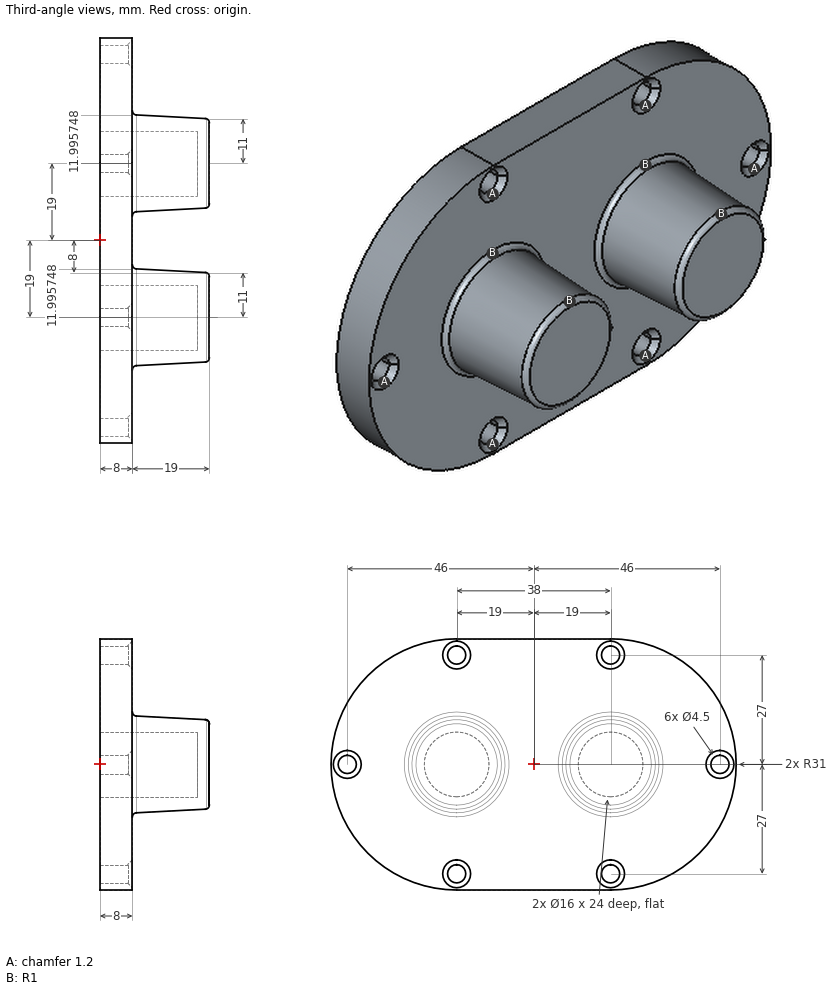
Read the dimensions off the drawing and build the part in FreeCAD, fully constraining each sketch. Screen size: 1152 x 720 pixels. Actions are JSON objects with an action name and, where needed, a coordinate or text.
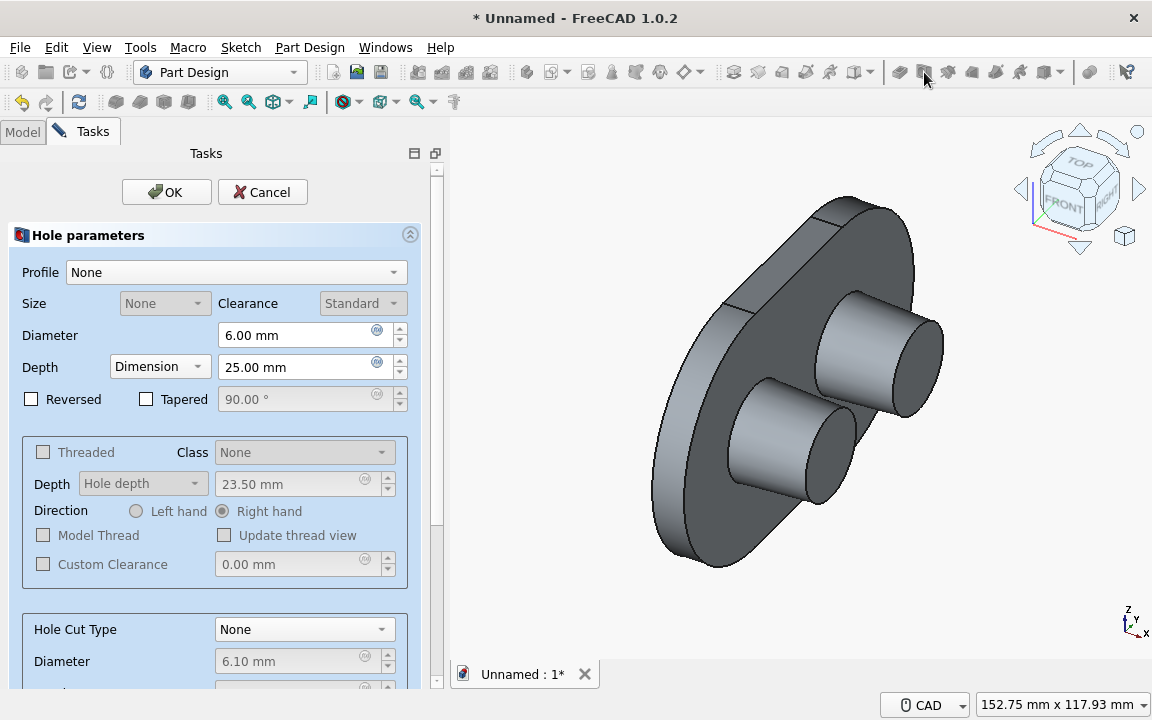
{"action": "triple_click", "coordinate": [305, 335]}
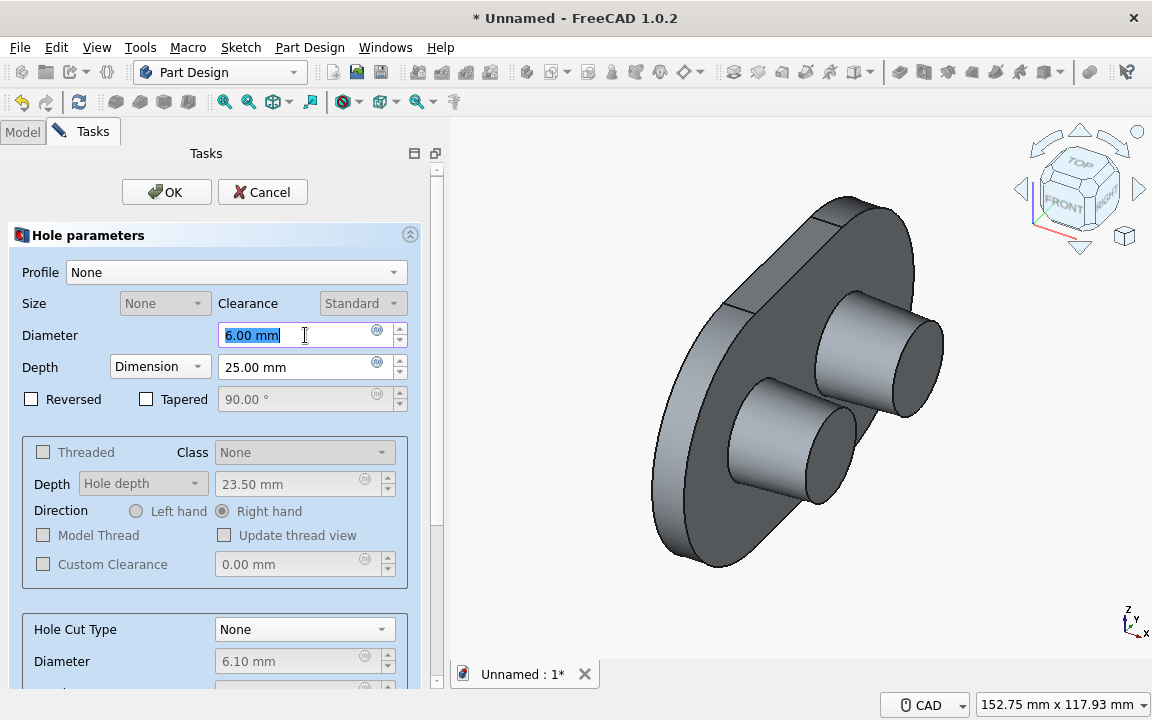
{"action": "type", "text": "16"}
{"action": "key", "text": "Tab"}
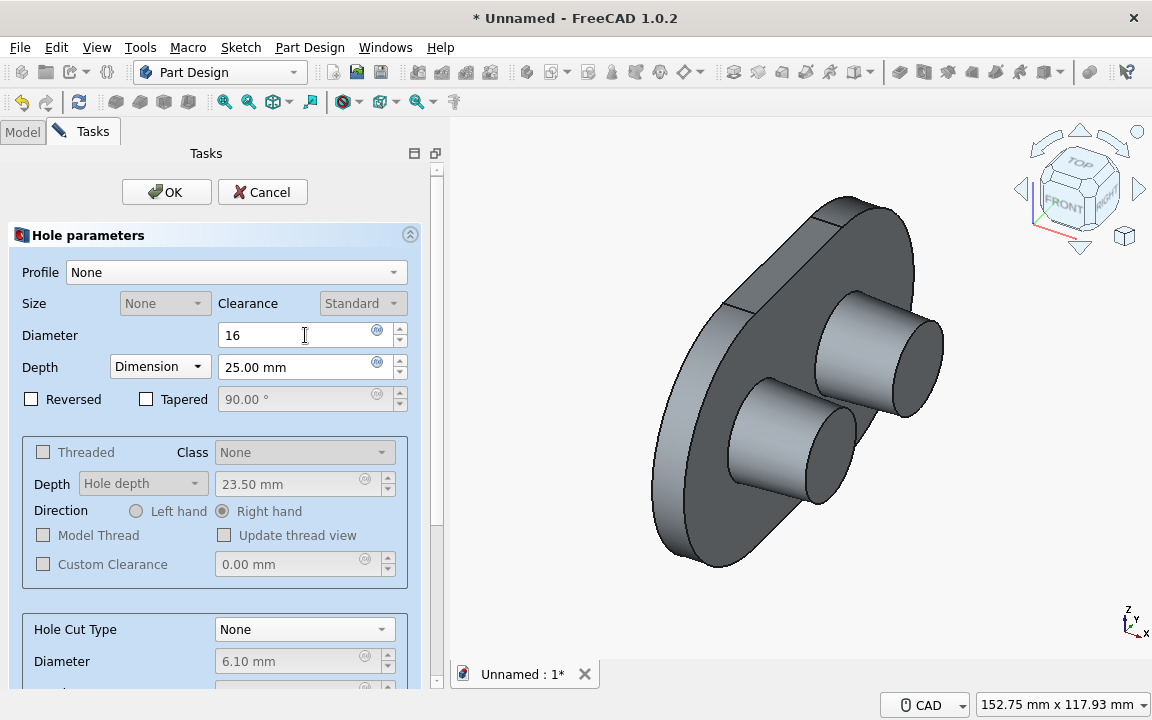
{"action": "triple_click", "coordinate": [305, 367]}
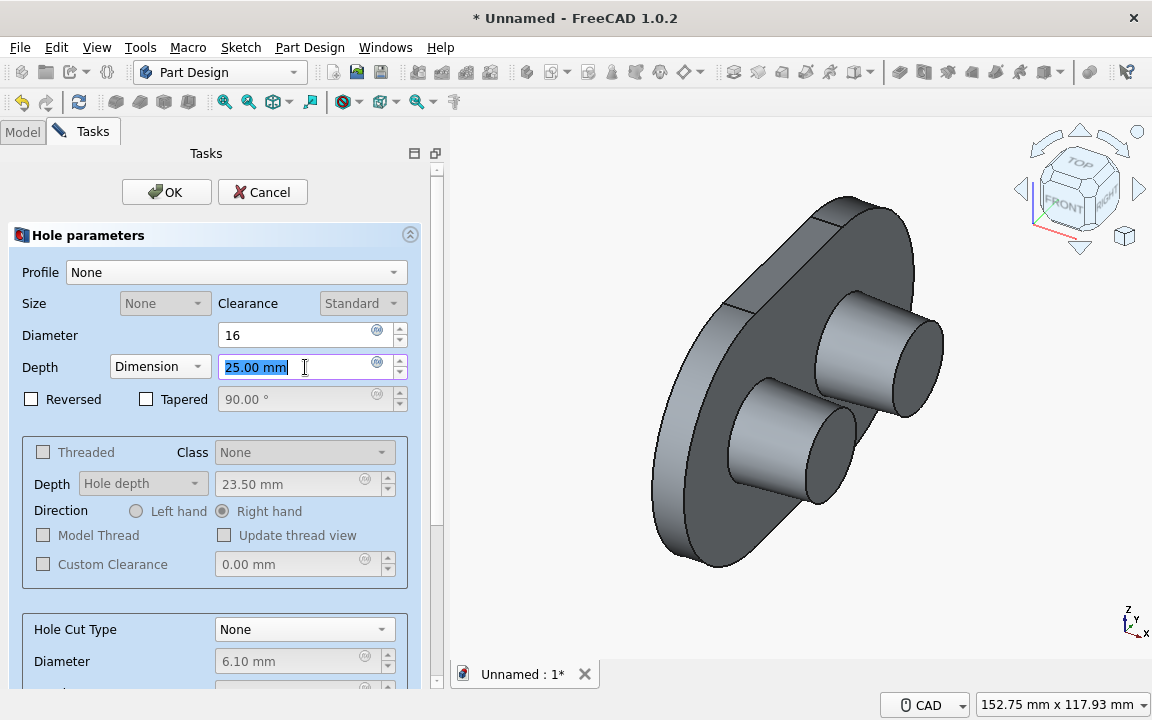
{"action": "type", "text": "24"}
{"action": "key", "text": "Tab"}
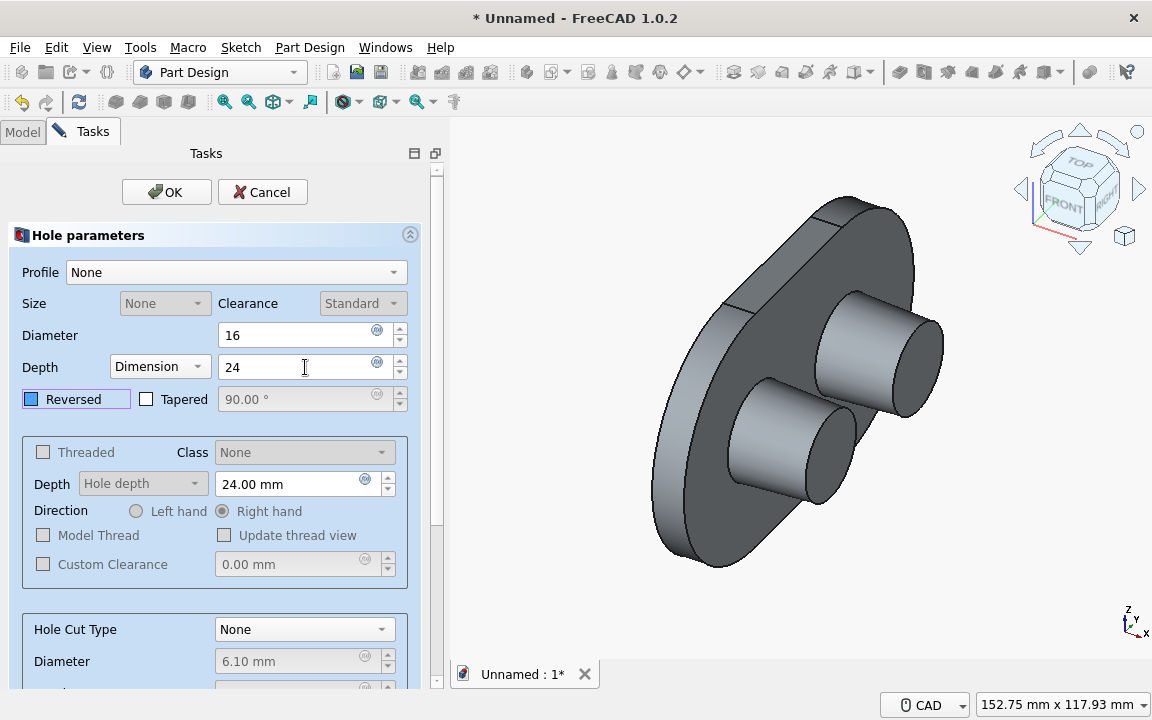
{"action": "left_click", "coordinate": [30, 399]}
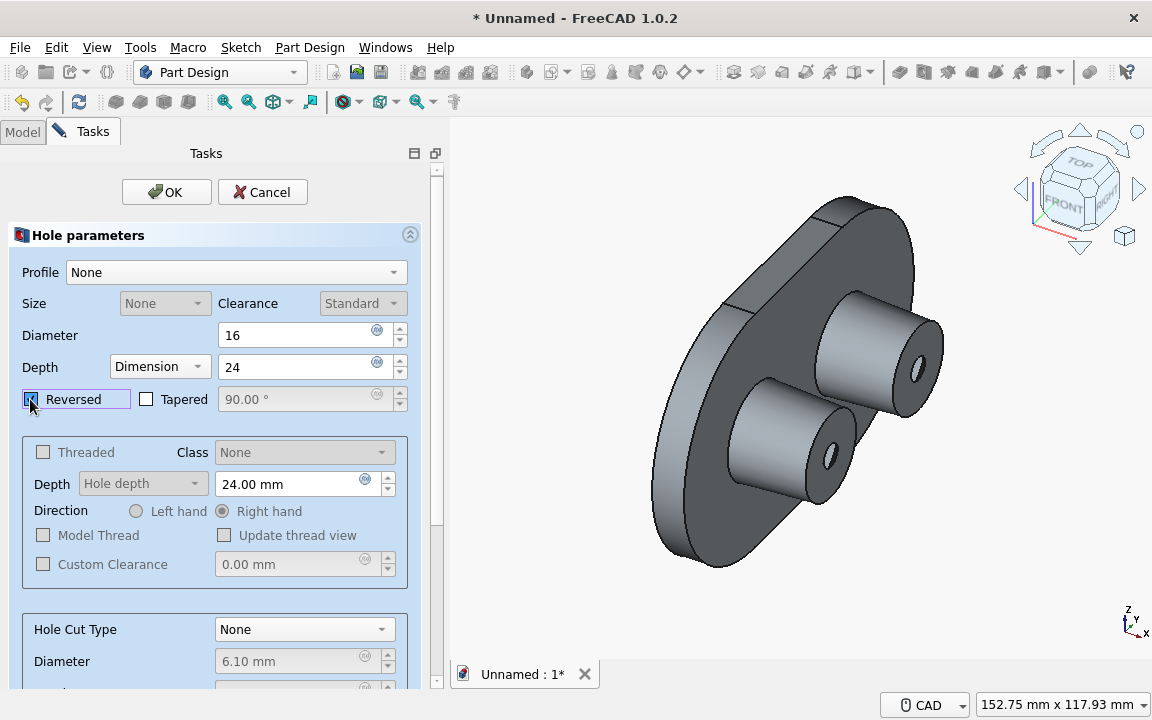
{"action": "scroll", "coordinate": [437, 426], "scroll_direction": "down", "scroll_amount": 4}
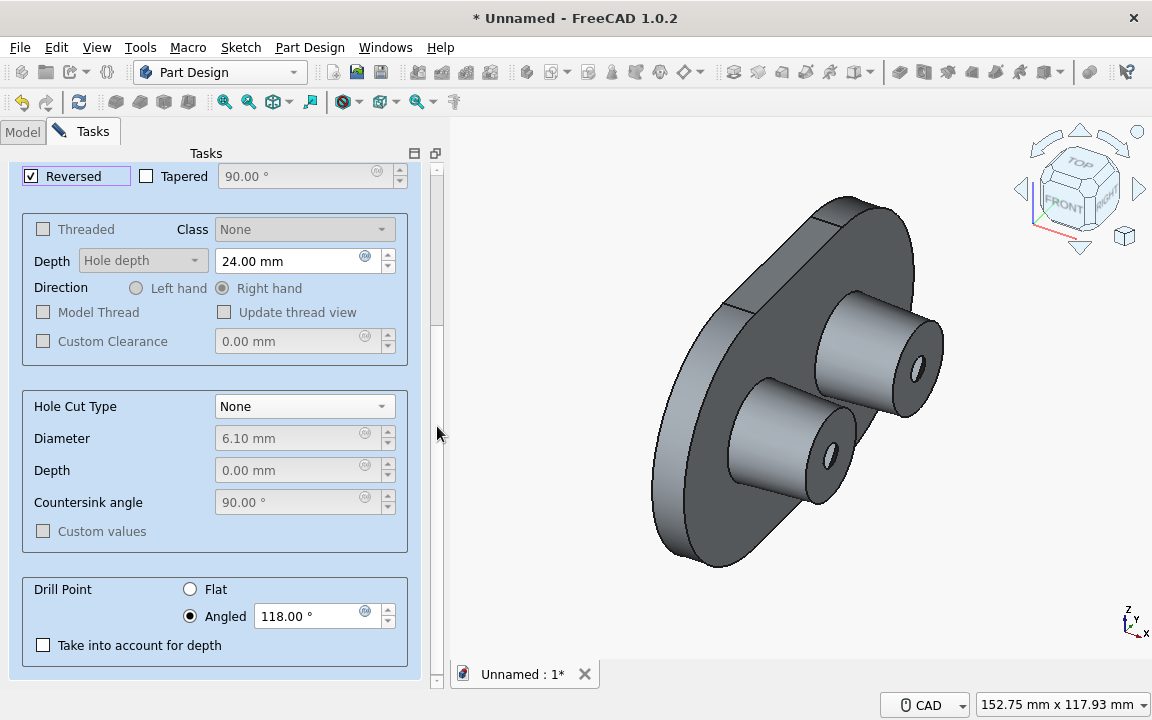
{"action": "left_click", "coordinate": [191, 589]}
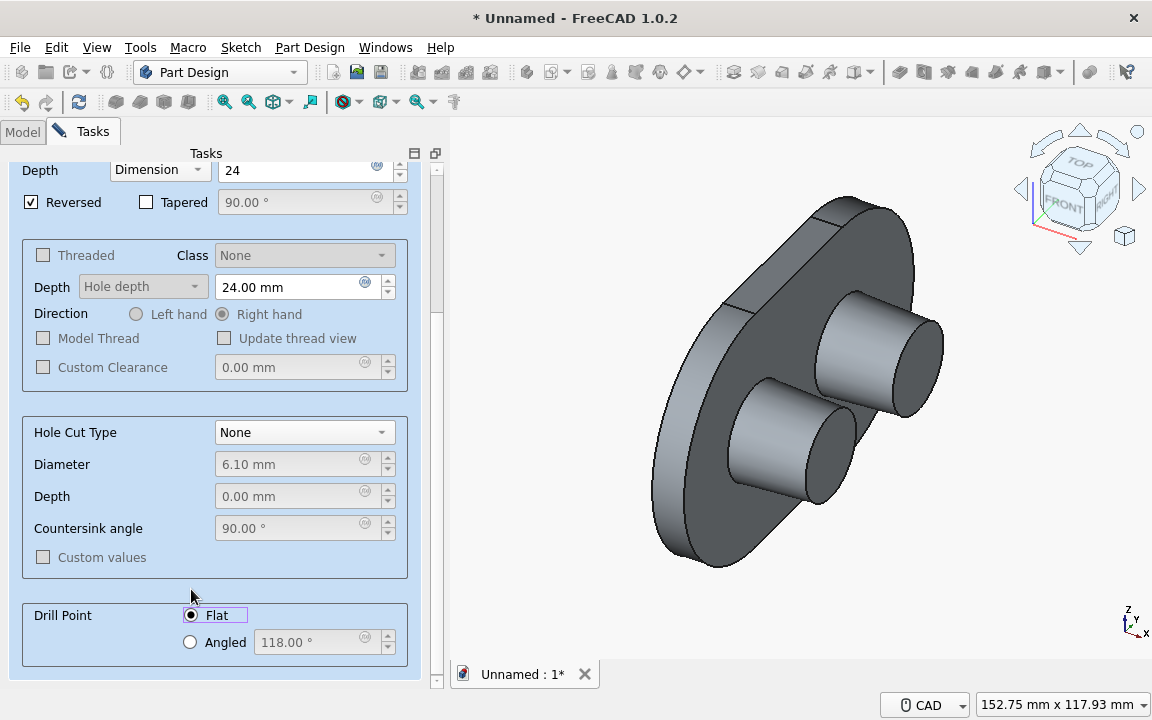
{"action": "scroll", "coordinate": [437, 426], "scroll_direction": "up", "scroll_amount": 5}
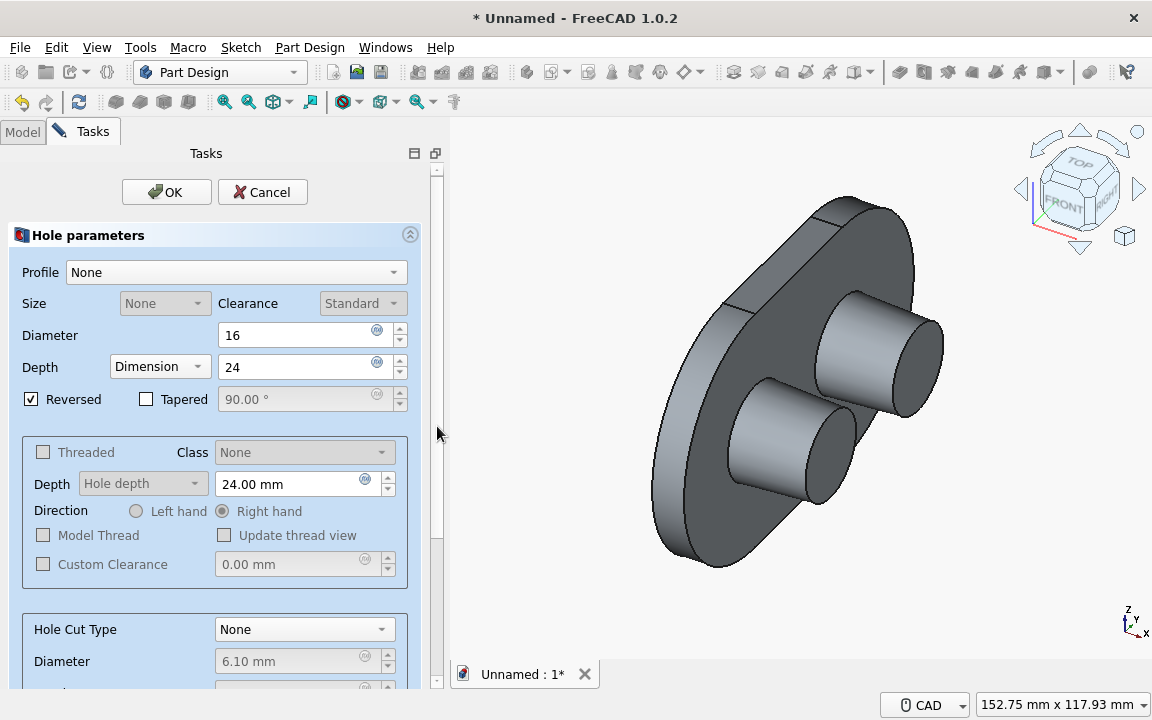
{"action": "left_click", "coordinate": [167, 192]}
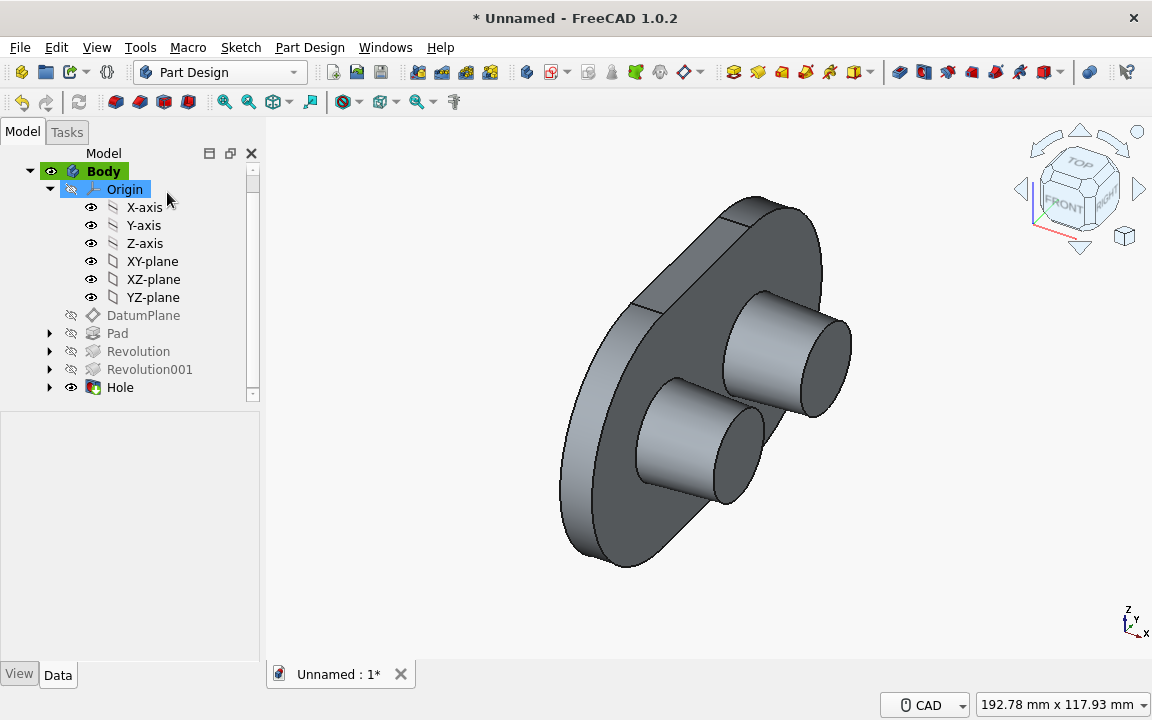
{"action": "left_click", "coordinate": [707, 320]}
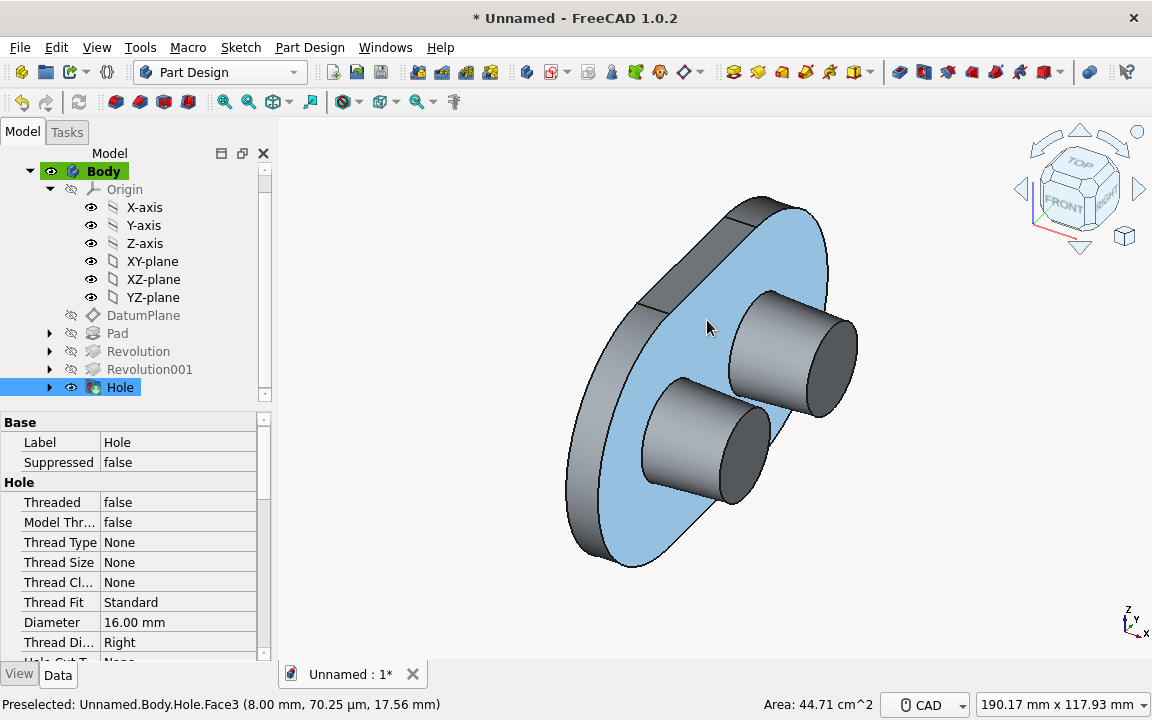
{"action": "left_click", "coordinate": [552, 72]}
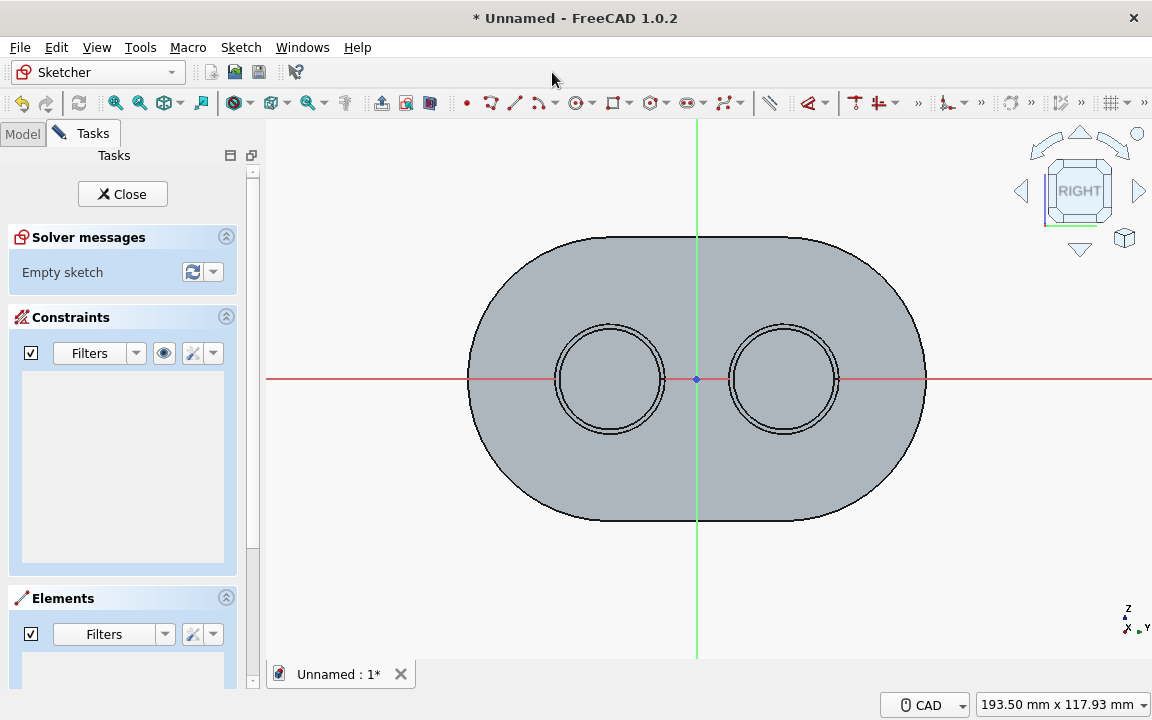
{"action": "left_click", "coordinate": [576, 104]}